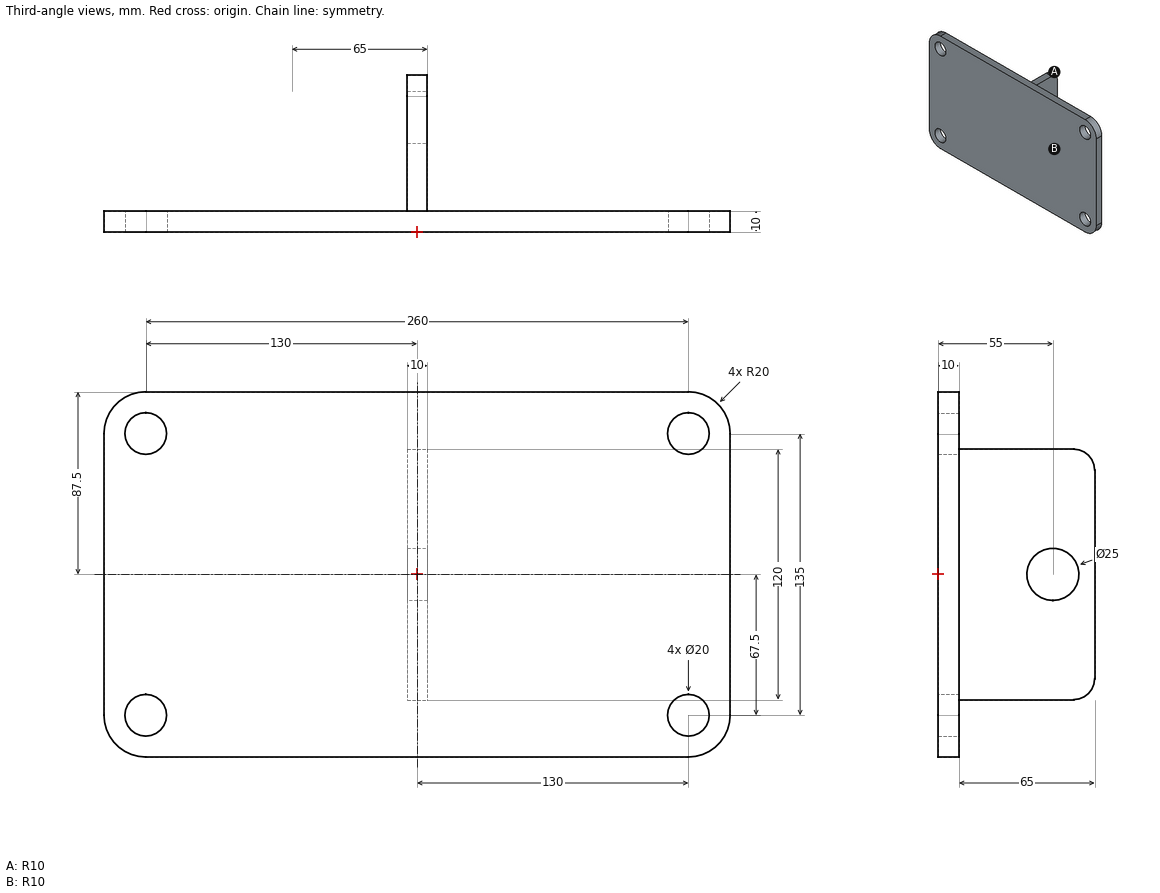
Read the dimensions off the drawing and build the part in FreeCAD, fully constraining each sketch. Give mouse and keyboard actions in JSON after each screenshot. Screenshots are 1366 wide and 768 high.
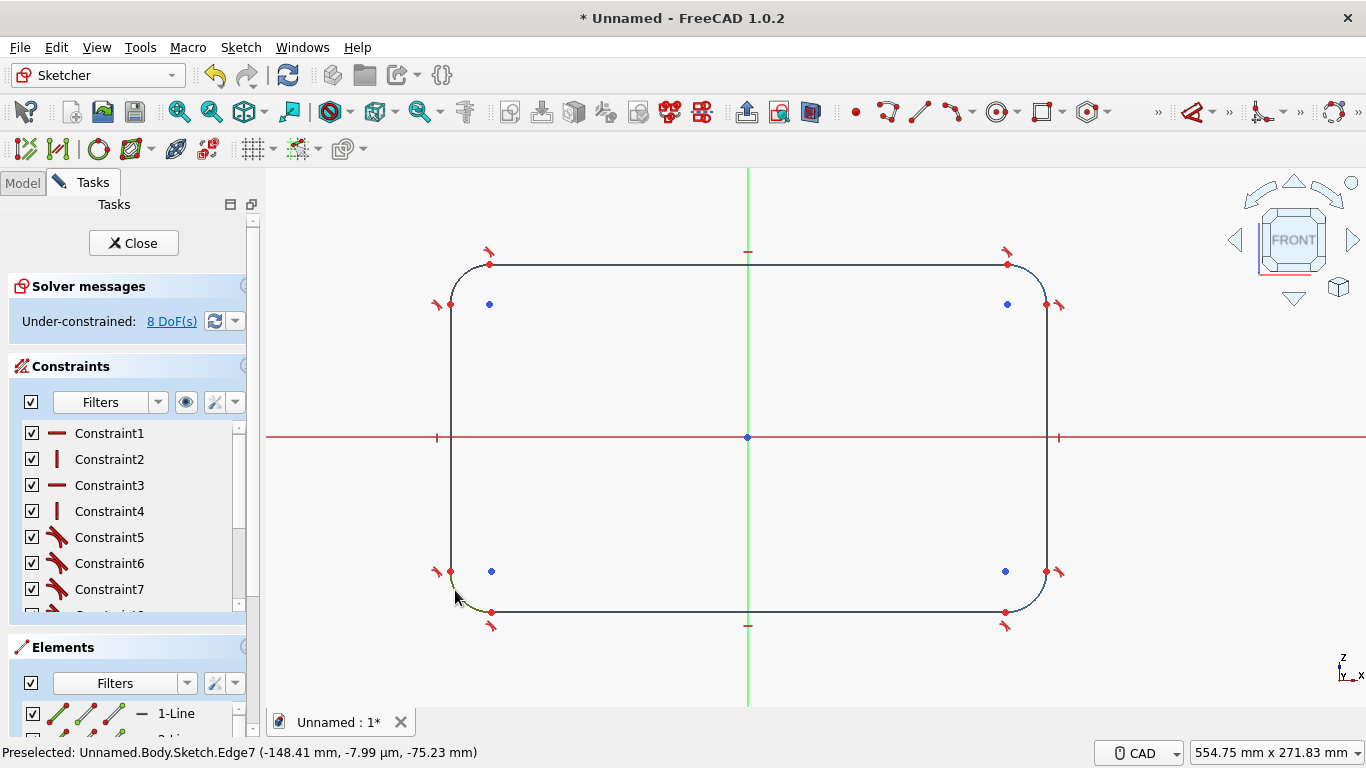
{"action": "left_click", "coordinate": [472, 269]}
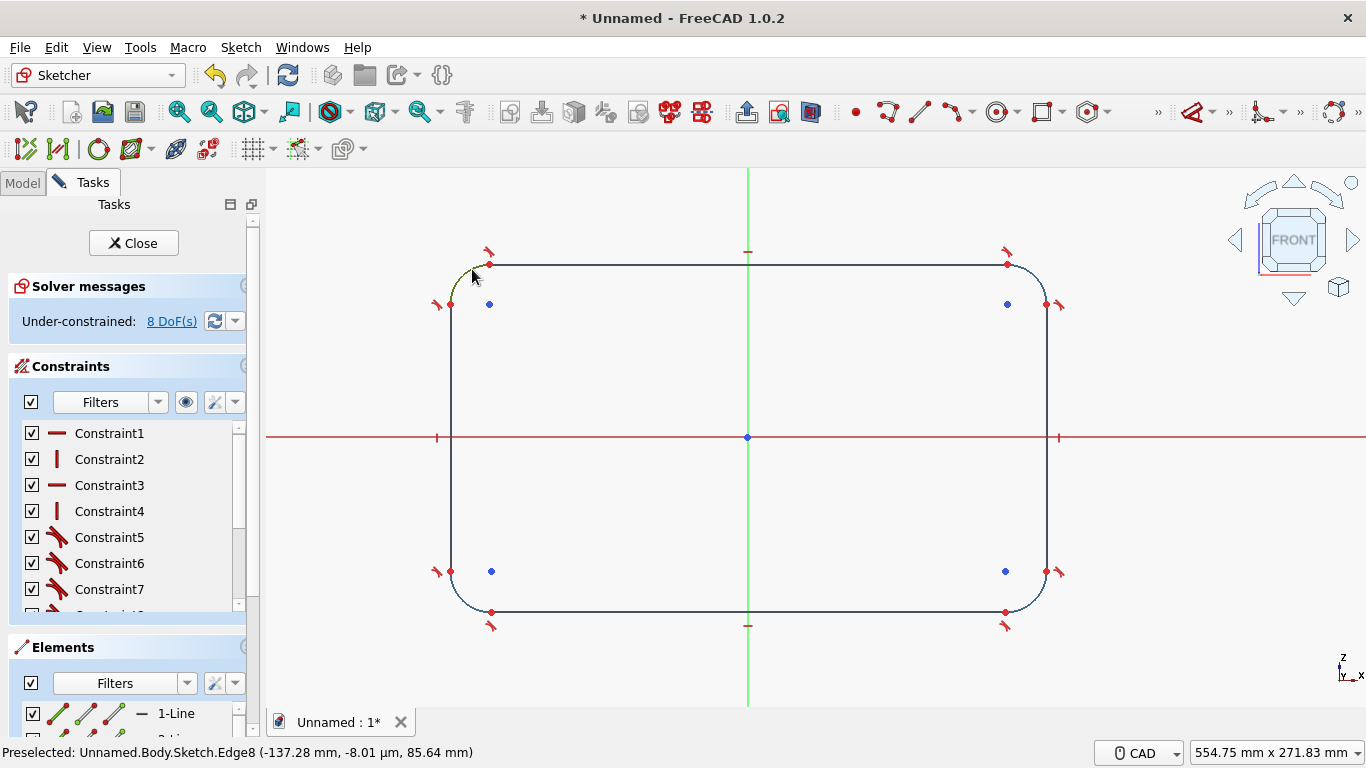
{"action": "key", "text": "e"}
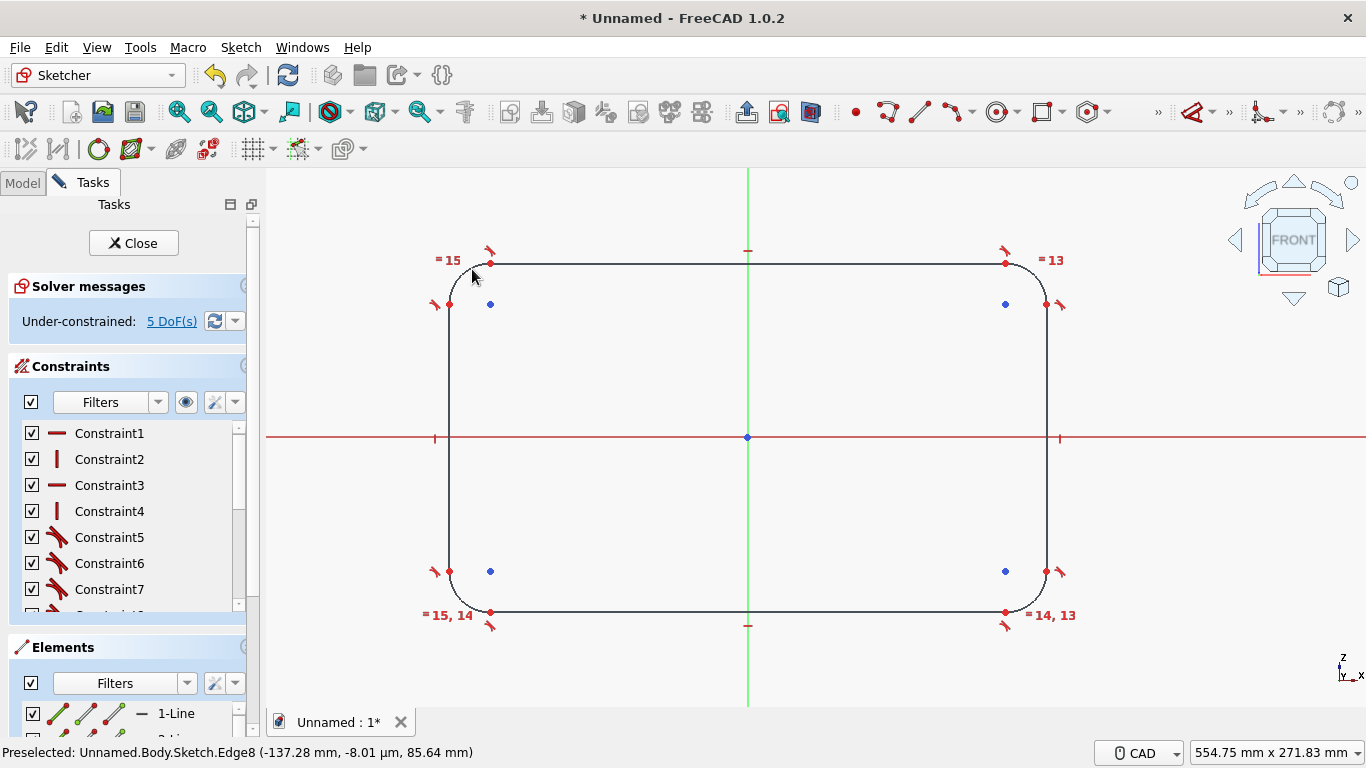
{"action": "left_click", "coordinate": [1192, 112]}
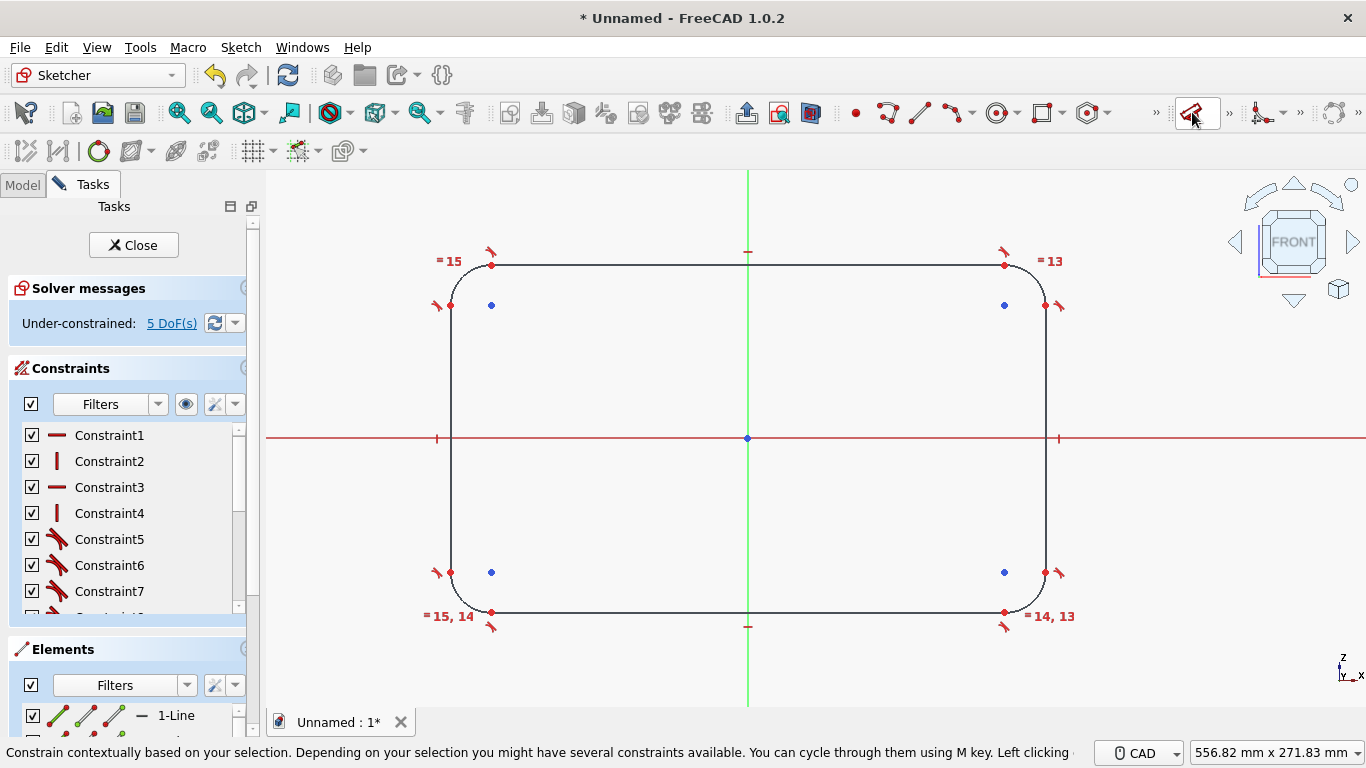
{"action": "left_click", "coordinate": [1041, 287]}
{"action": "left_click", "coordinate": [1069, 272]}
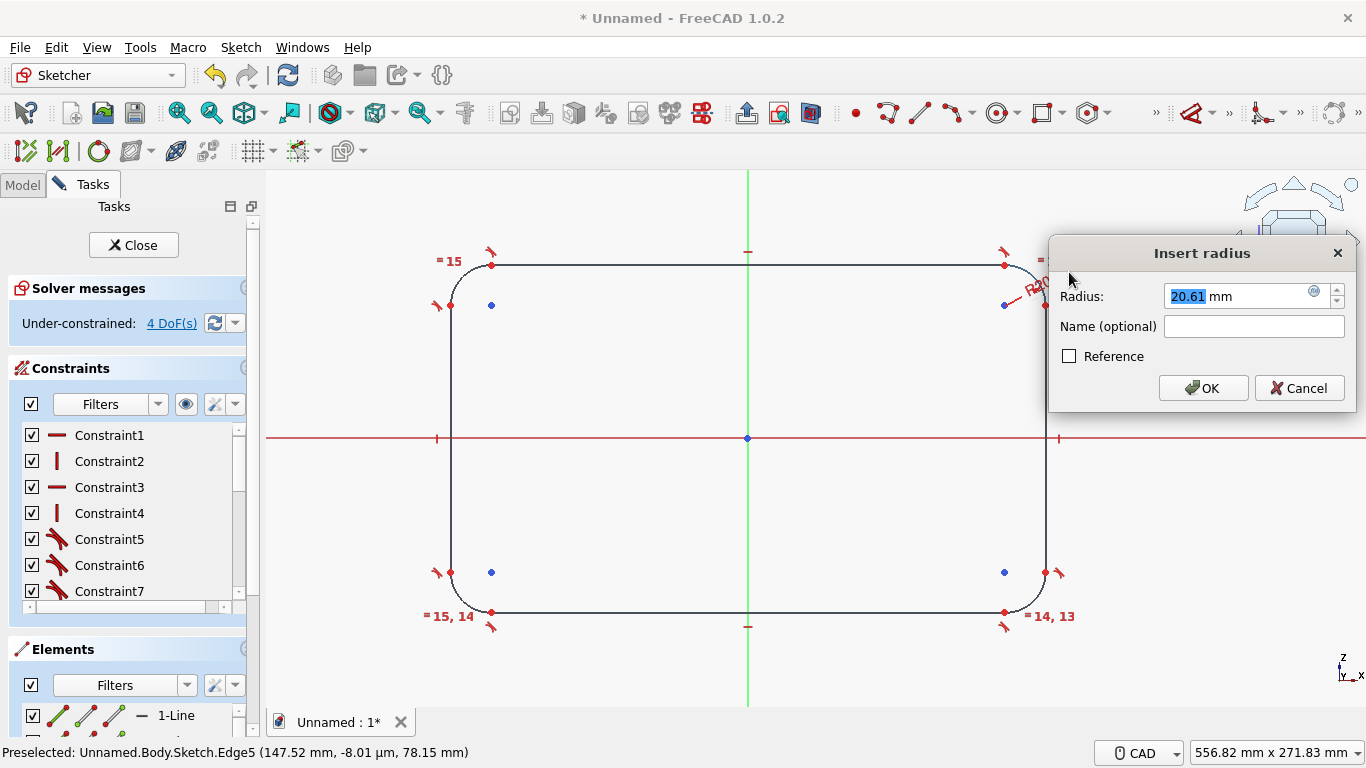
{"action": "type", "text": "20"}
{"action": "key", "text": "Return"}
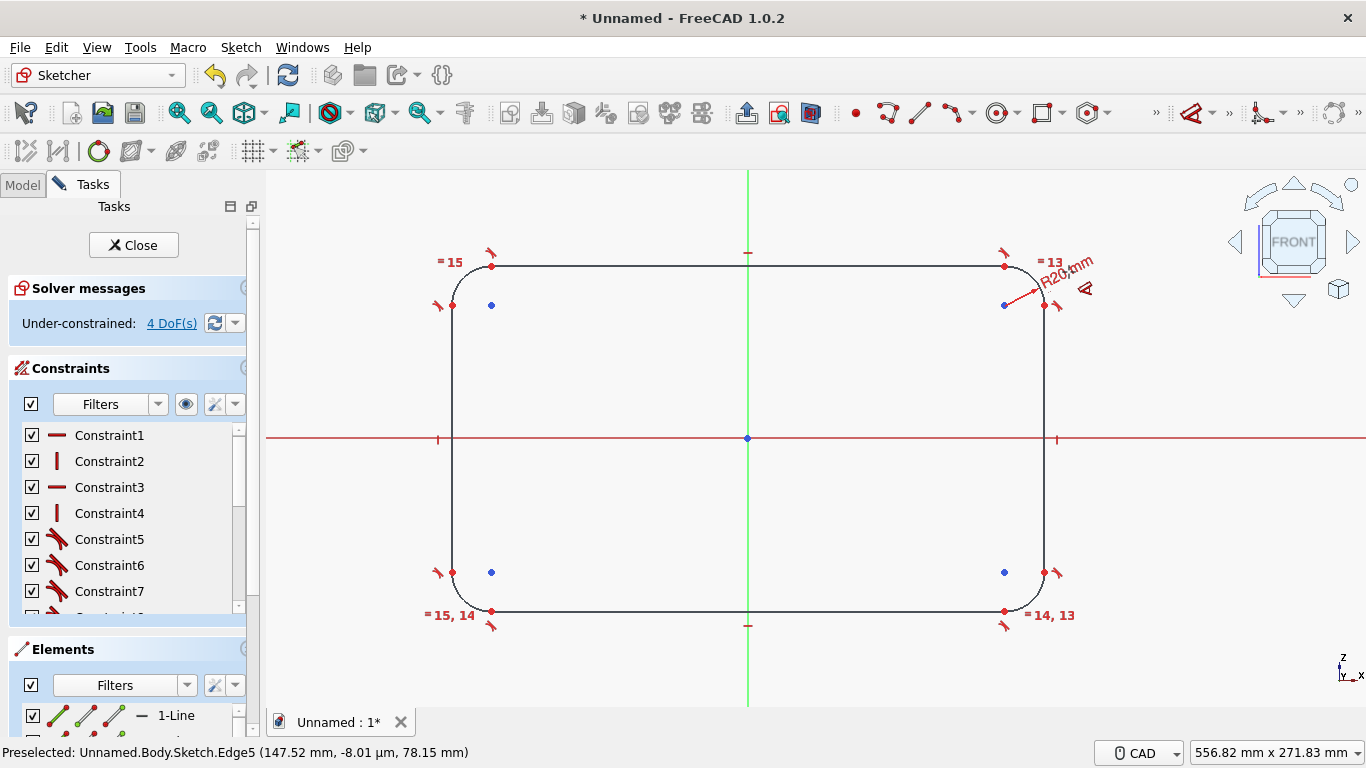
{"action": "left_click", "coordinate": [646, 266]}
{"action": "left_click", "coordinate": [630, 232]}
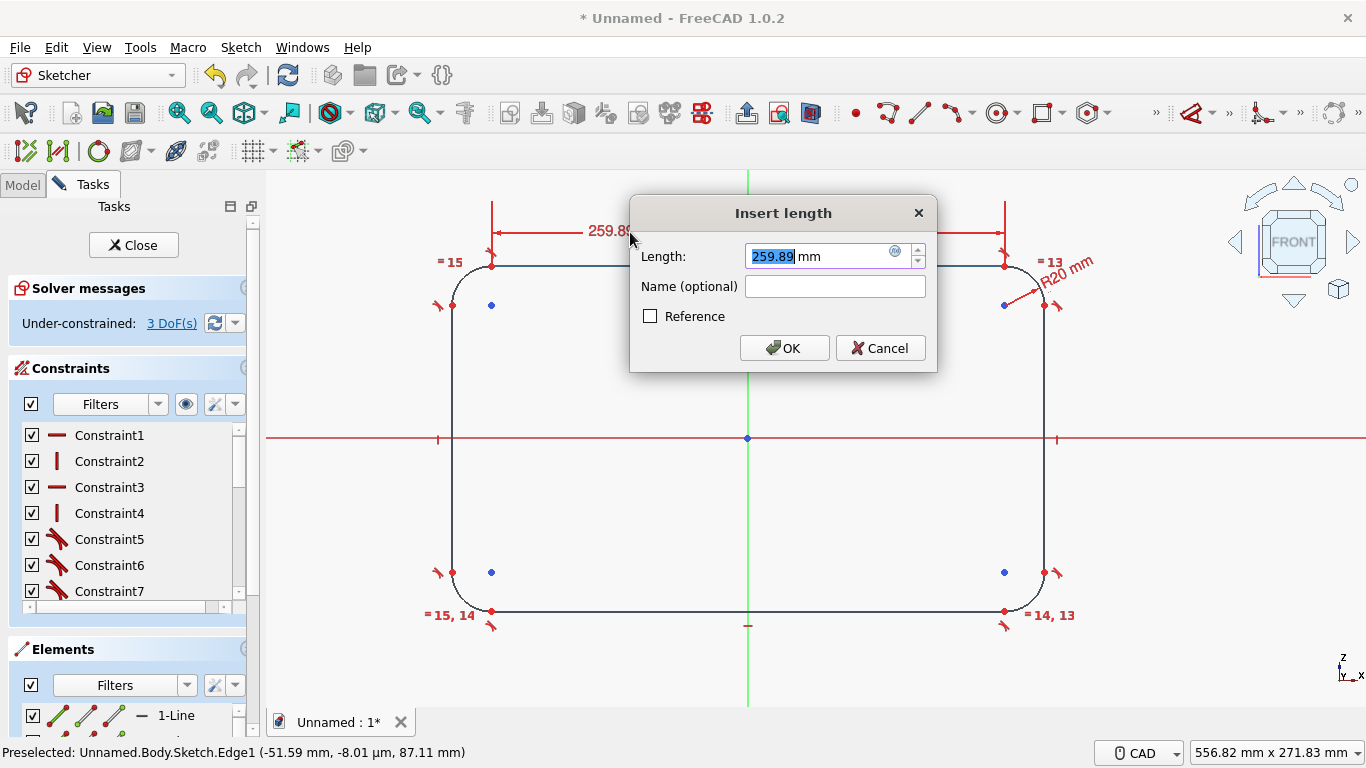
{"action": "type", "text": "260"}
{"action": "key", "text": "Return"}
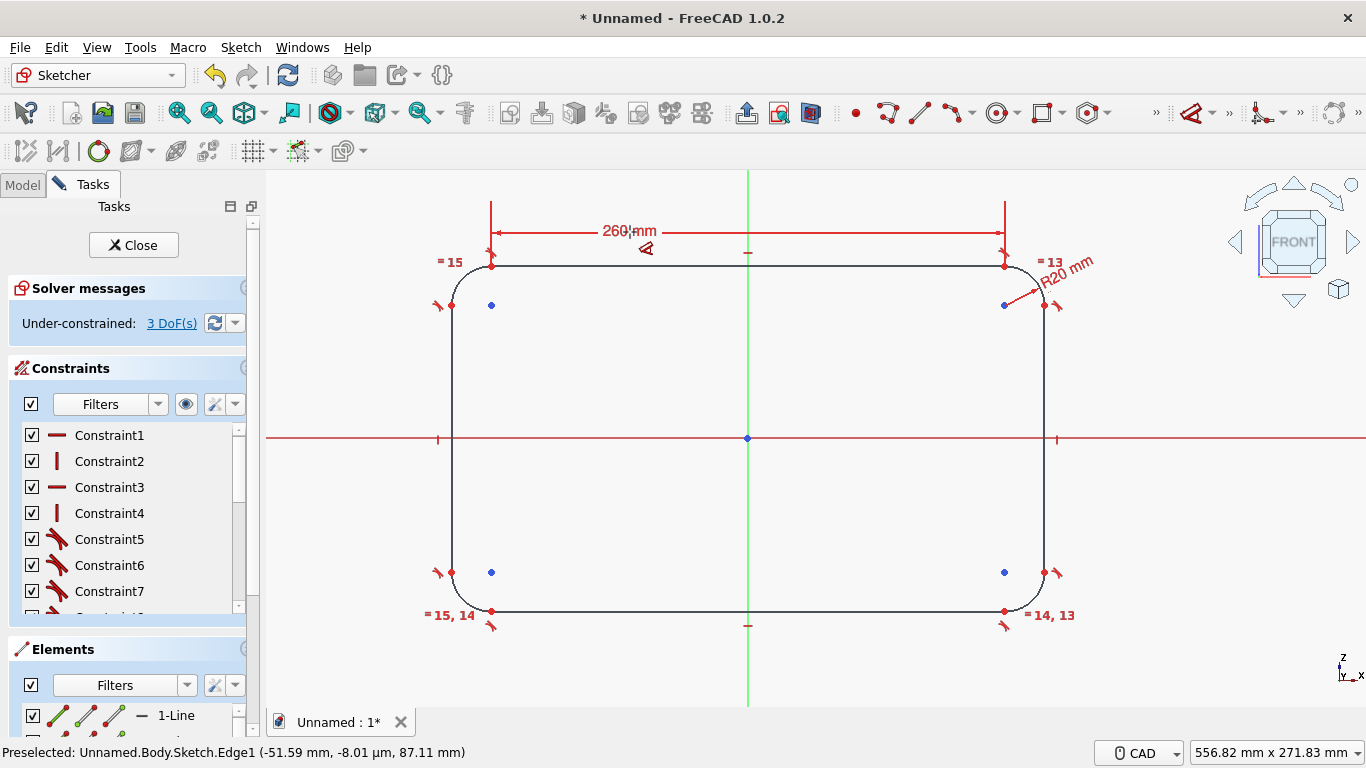
{"action": "left_click", "coordinate": [1044, 386]}
{"action": "left_click", "coordinate": [1078, 378]}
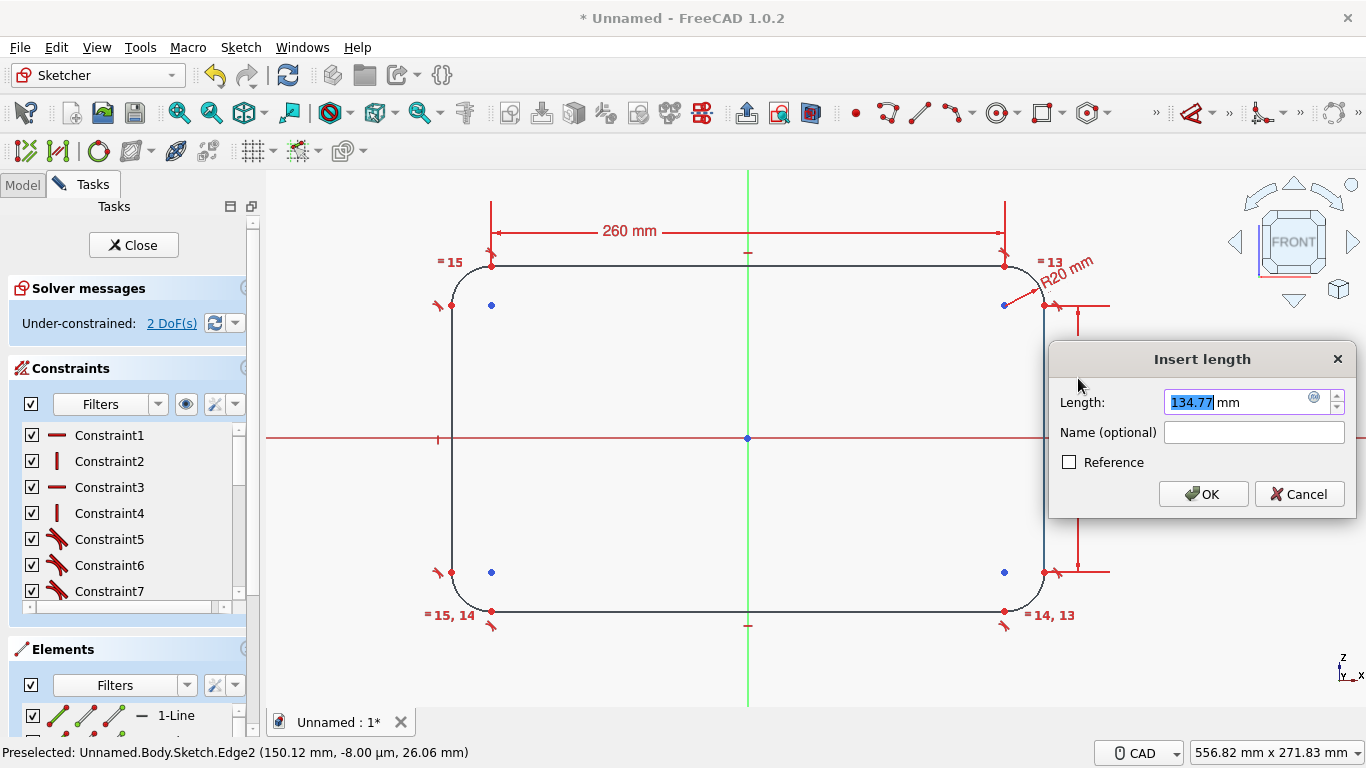
{"action": "type", "text": "135"}
{"action": "key", "text": "Return"}